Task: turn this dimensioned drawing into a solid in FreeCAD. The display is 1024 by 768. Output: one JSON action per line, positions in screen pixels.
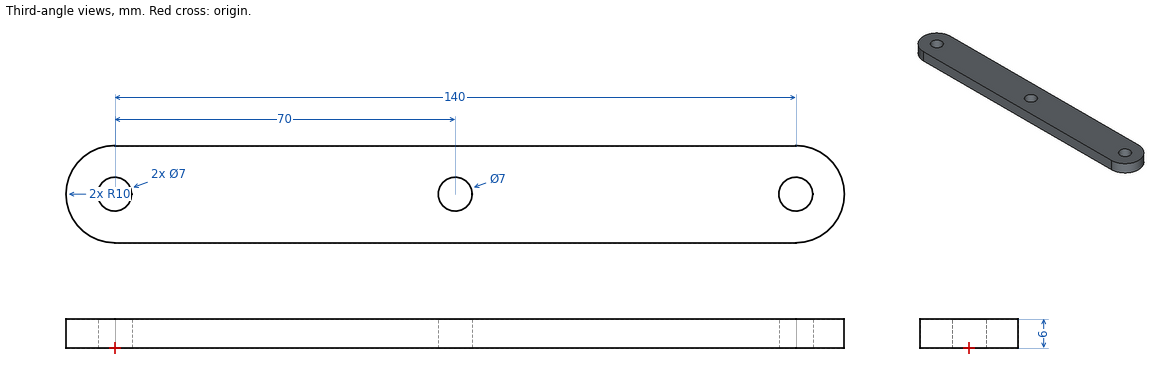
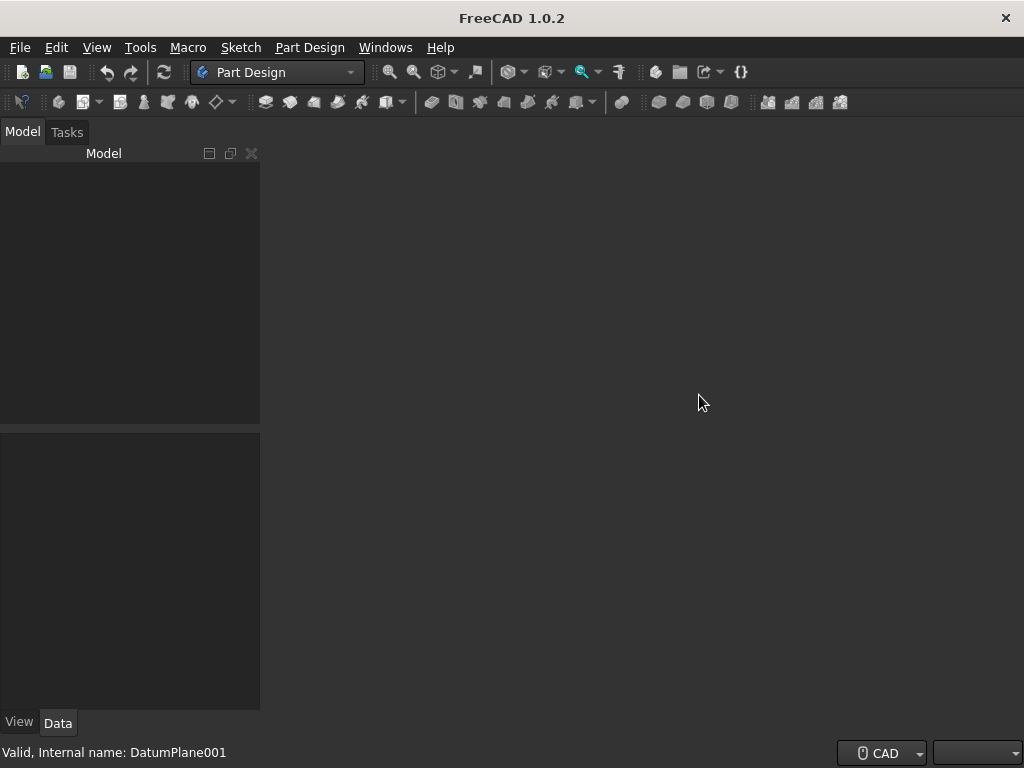
{"action": "left_click", "coordinate": [22, 72]}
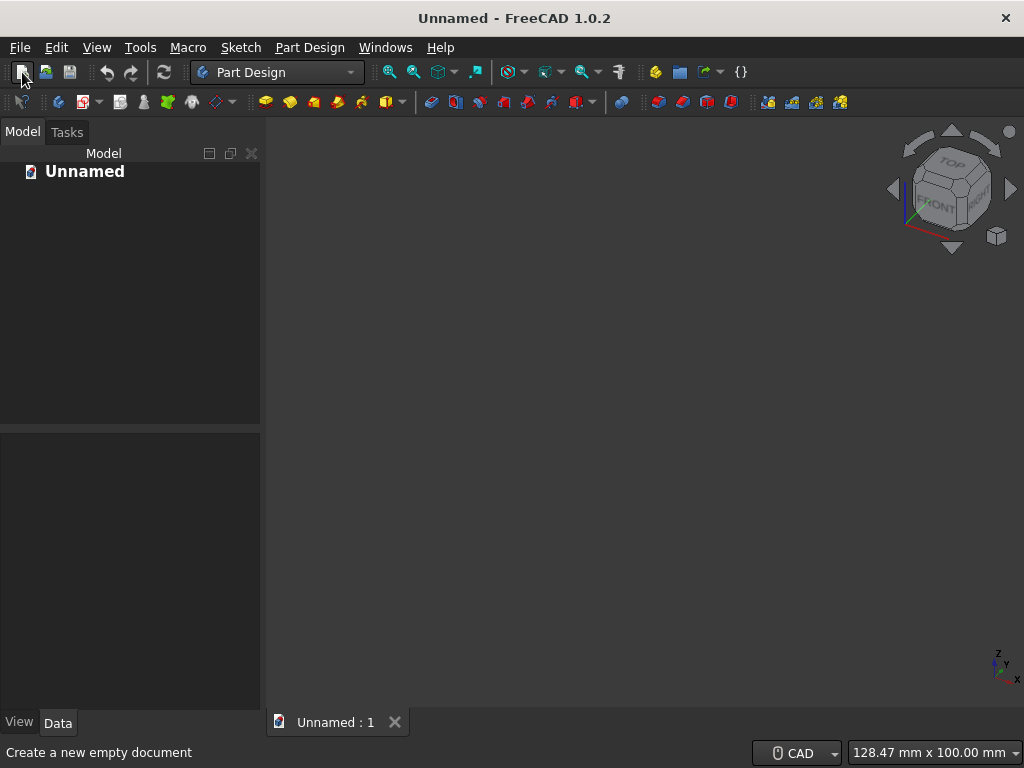
{"action": "left_click", "coordinate": [84, 102]}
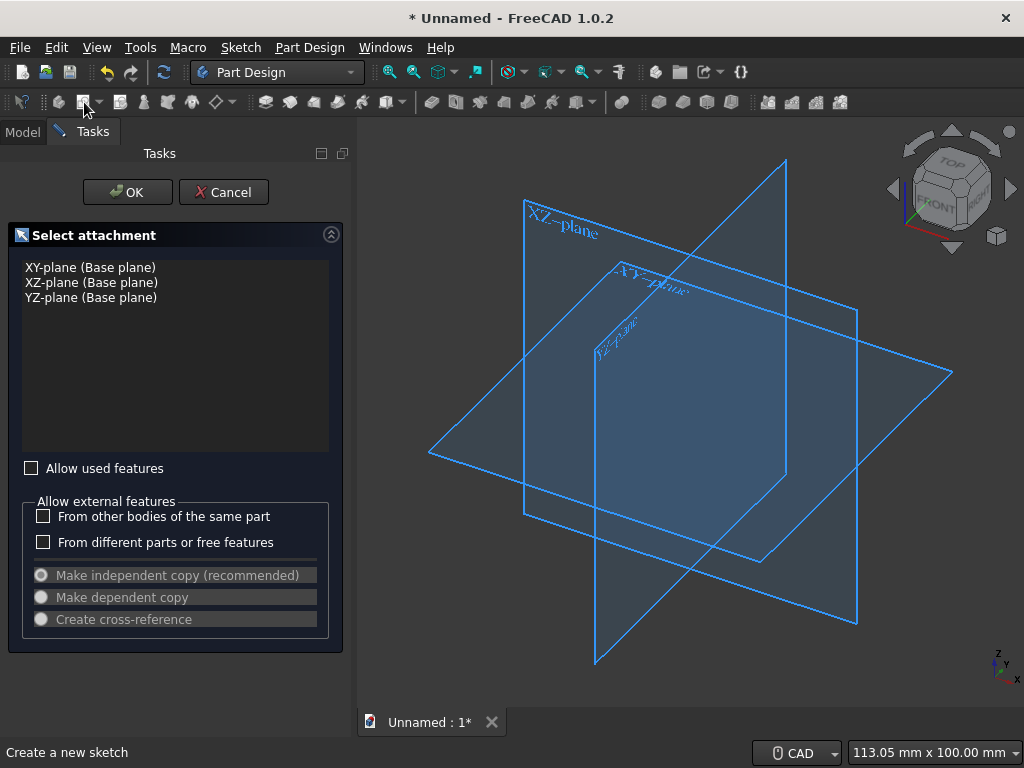
{"action": "left_click", "coordinate": [82, 268]}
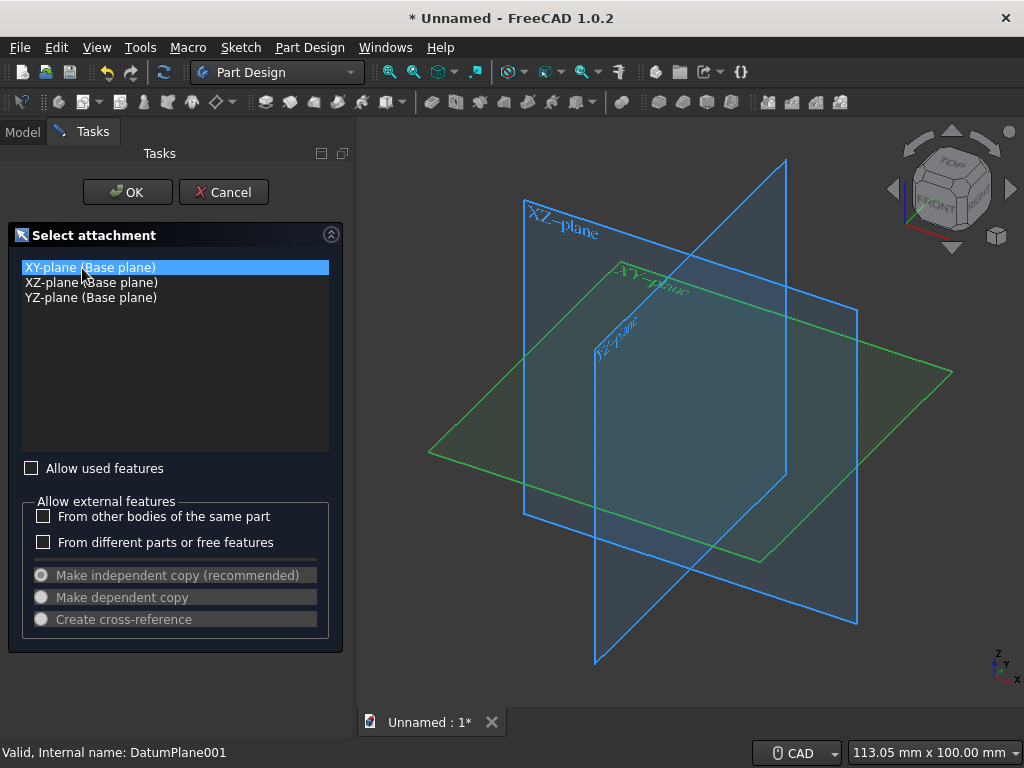
{"action": "left_click", "coordinate": [128, 192]}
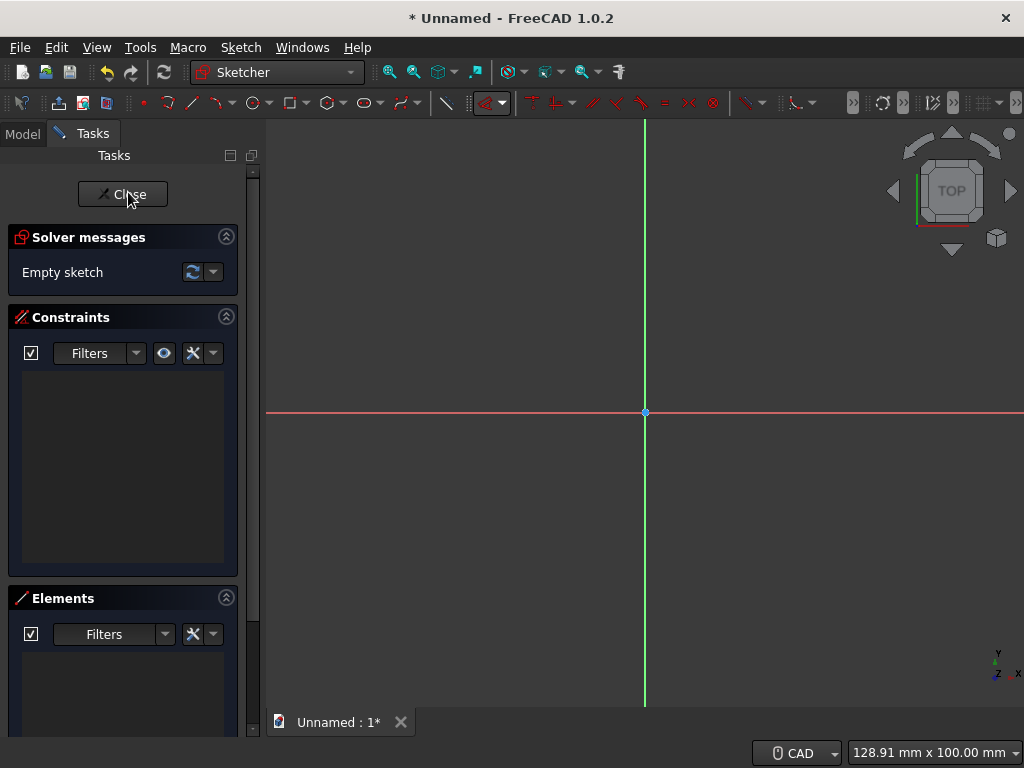
{"action": "scroll", "coordinate": [297, 413], "scroll_direction": "down", "scroll_amount": 5}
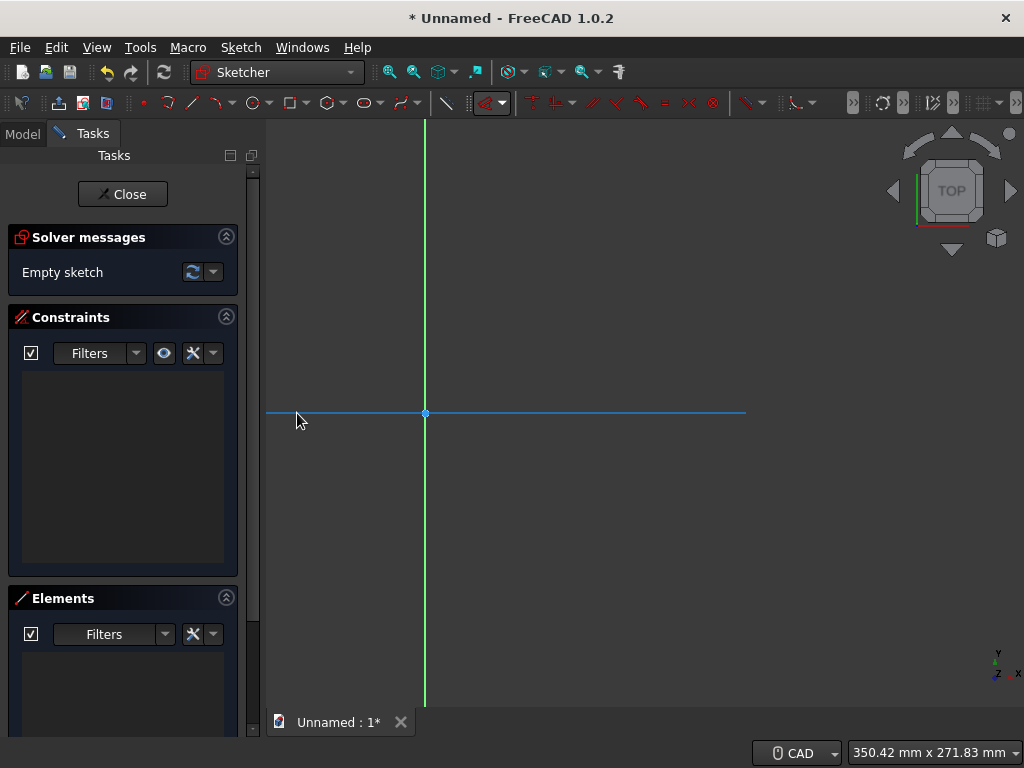
{"action": "left_click", "coordinate": [364, 104]}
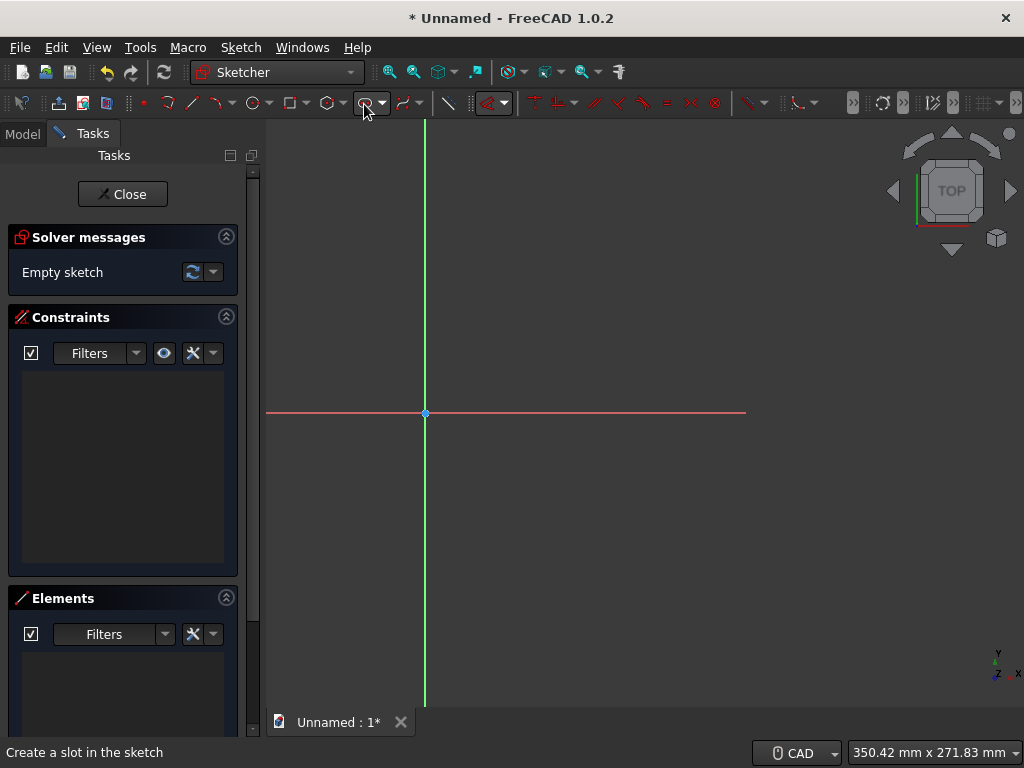
{"action": "left_click", "coordinate": [425, 413]}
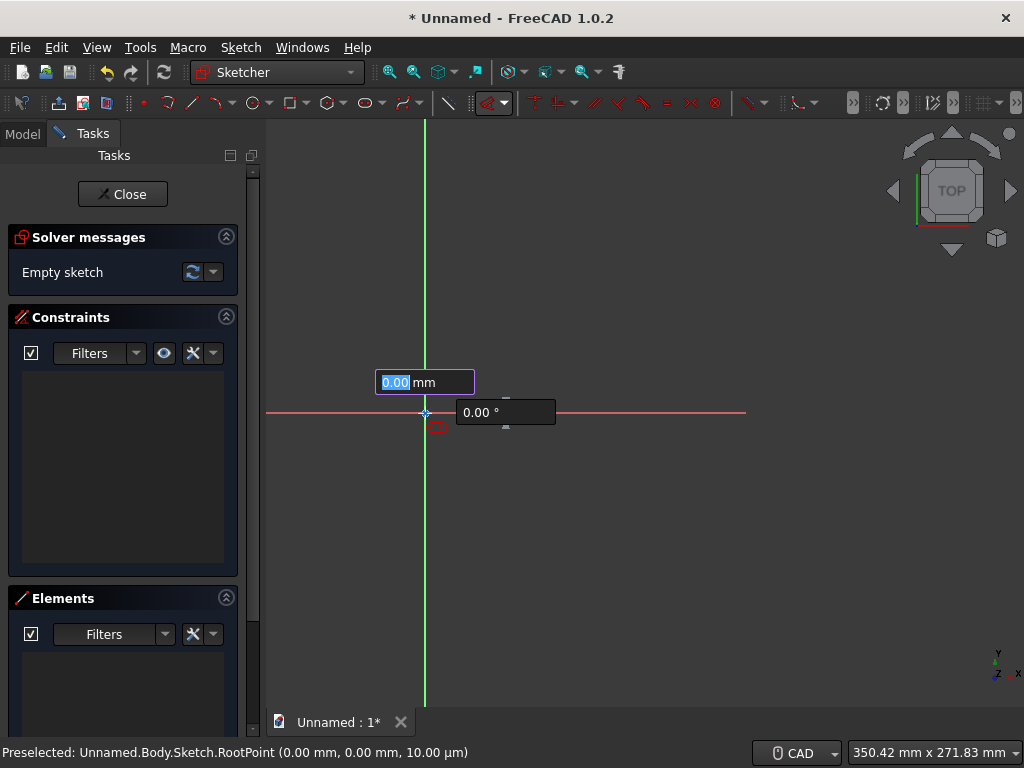
{"action": "left_click", "coordinate": [728, 404]}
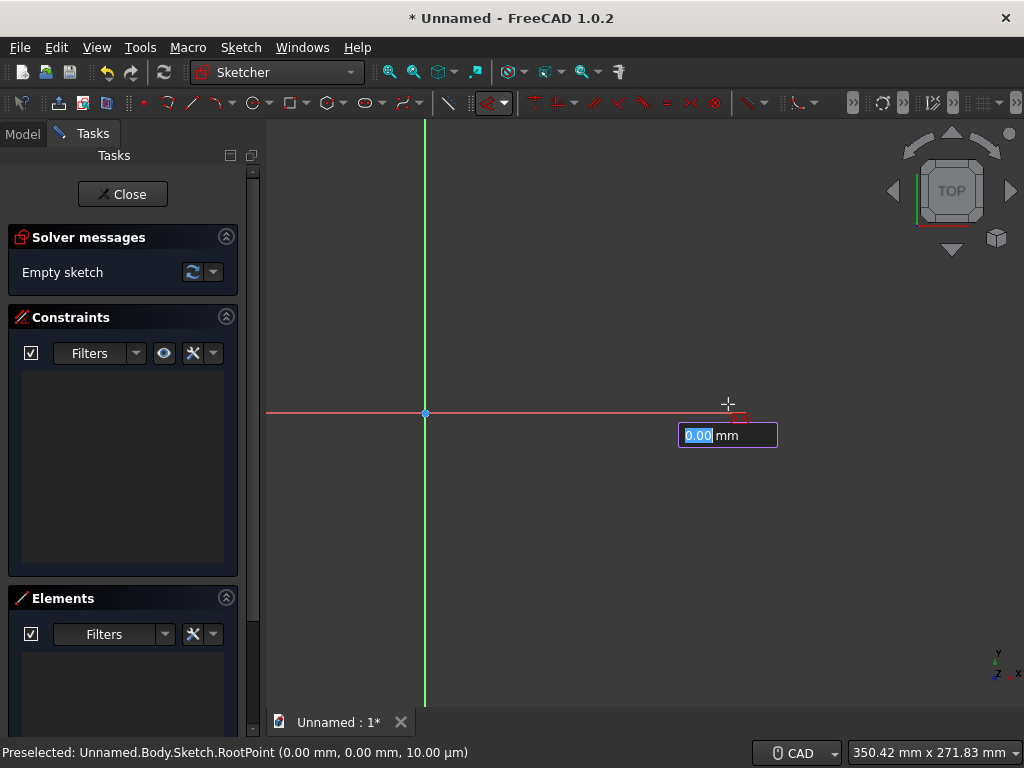
{"action": "left_click", "coordinate": [576, 392]}
{"action": "key", "text": "Escape"}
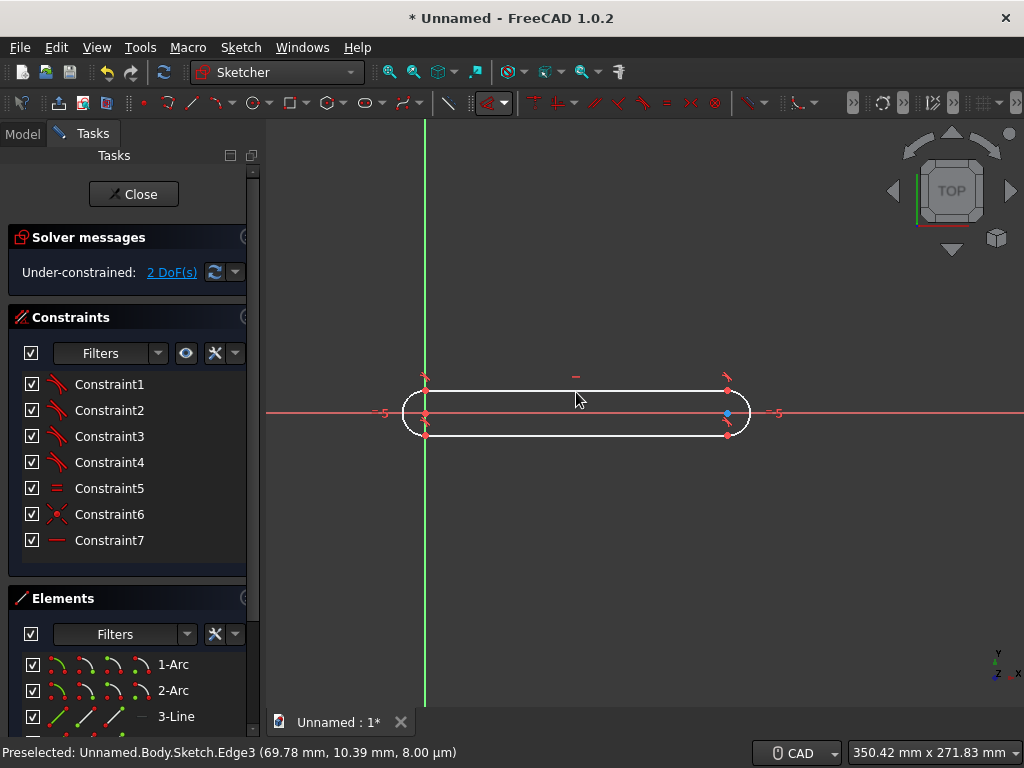
{"action": "scroll", "coordinate": [407, 400], "scroll_direction": "up", "scroll_amount": 4}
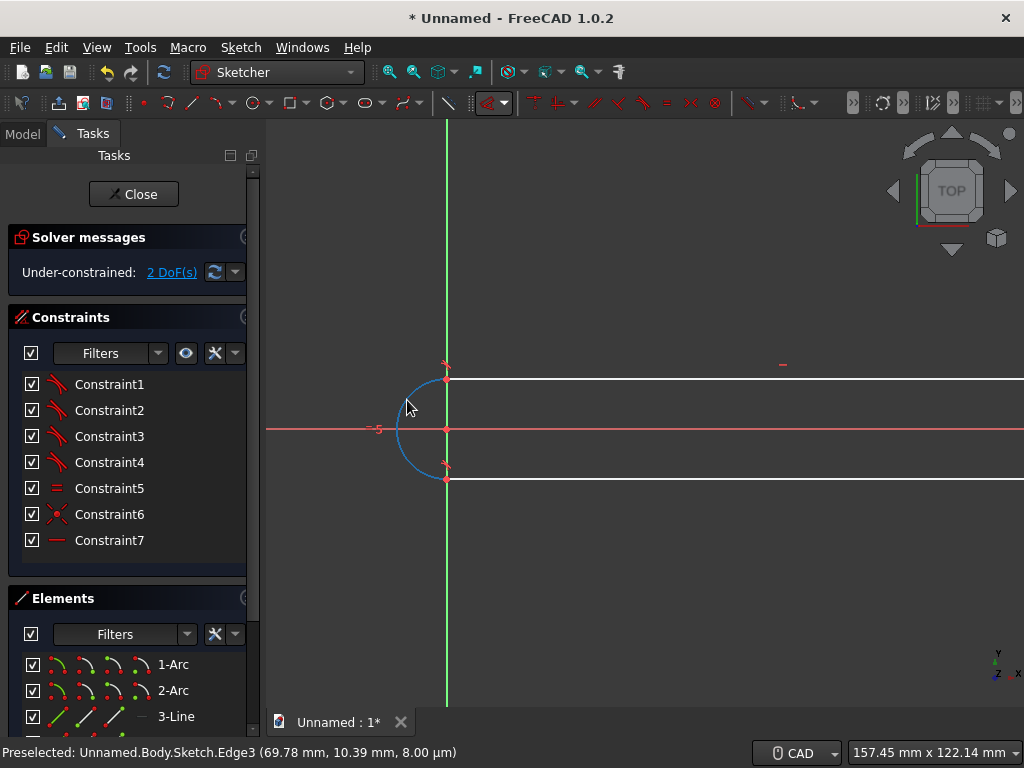
{"action": "left_click", "coordinate": [406, 400]}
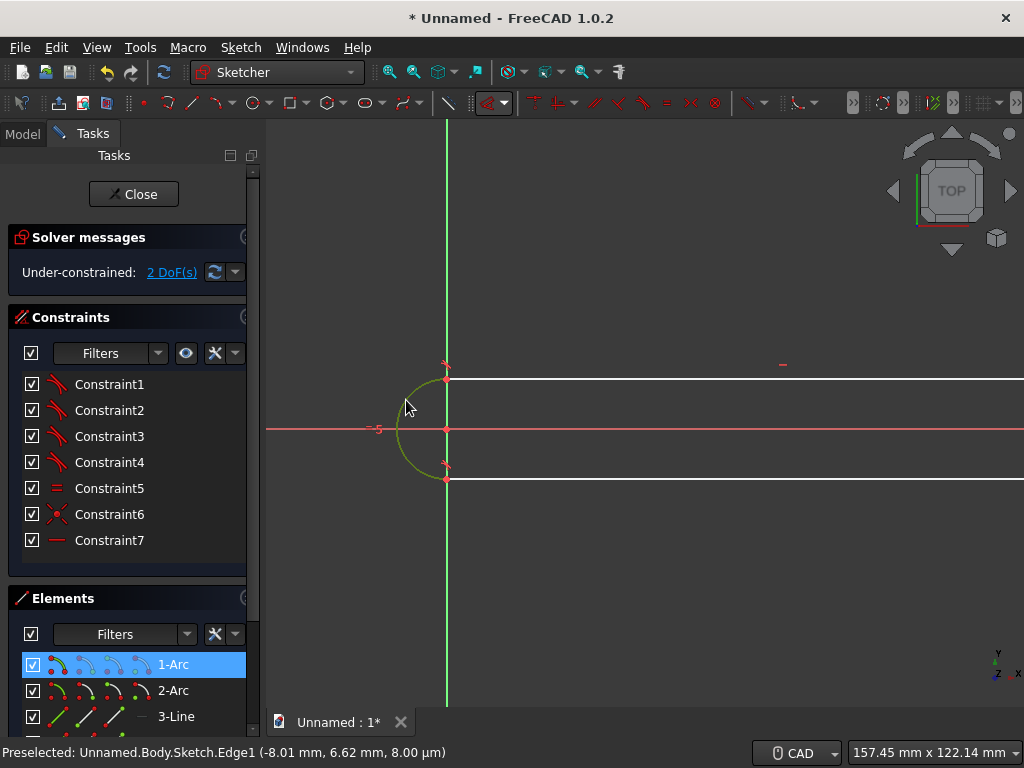
{"action": "left_click", "coordinate": [506, 104]}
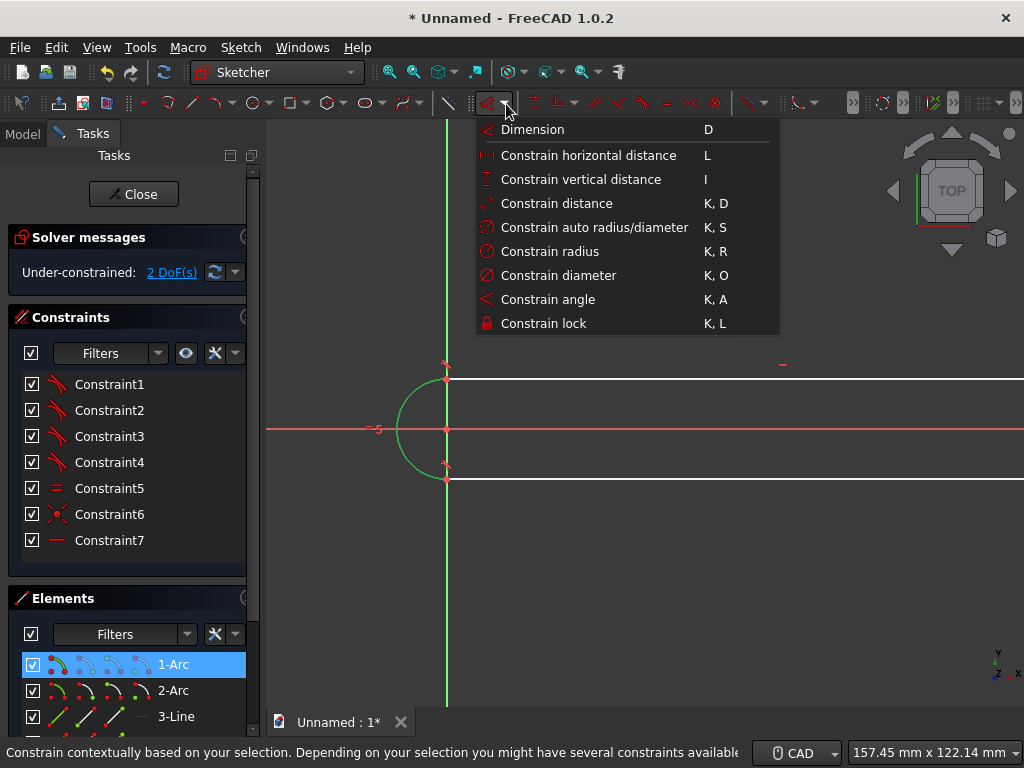
{"action": "left_click", "coordinate": [628, 251]}